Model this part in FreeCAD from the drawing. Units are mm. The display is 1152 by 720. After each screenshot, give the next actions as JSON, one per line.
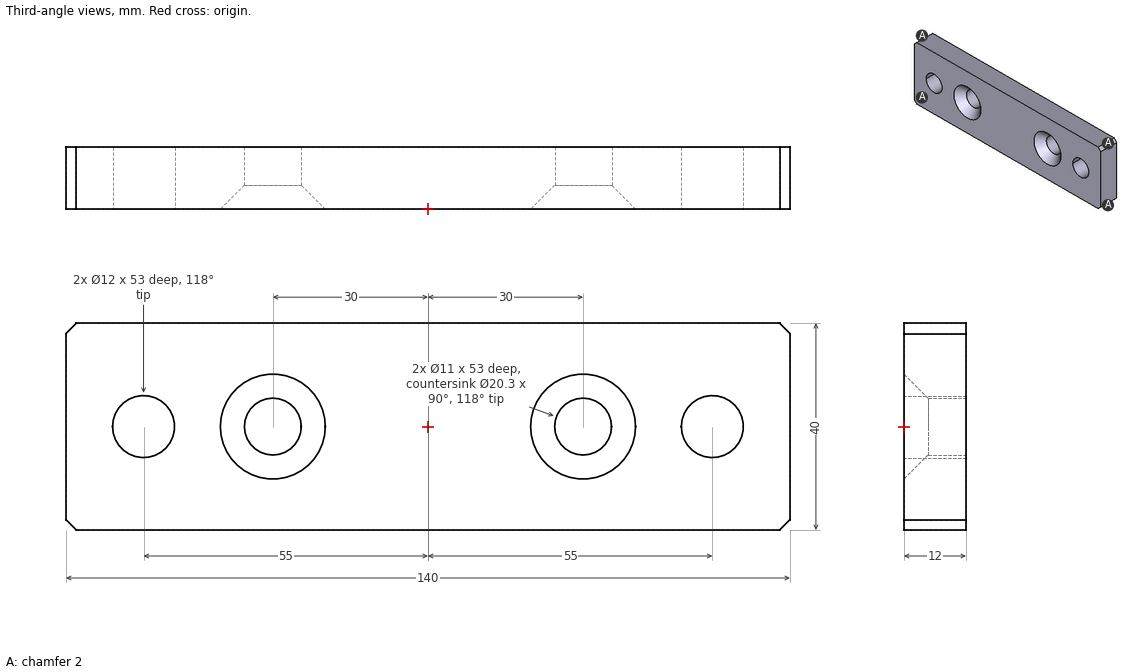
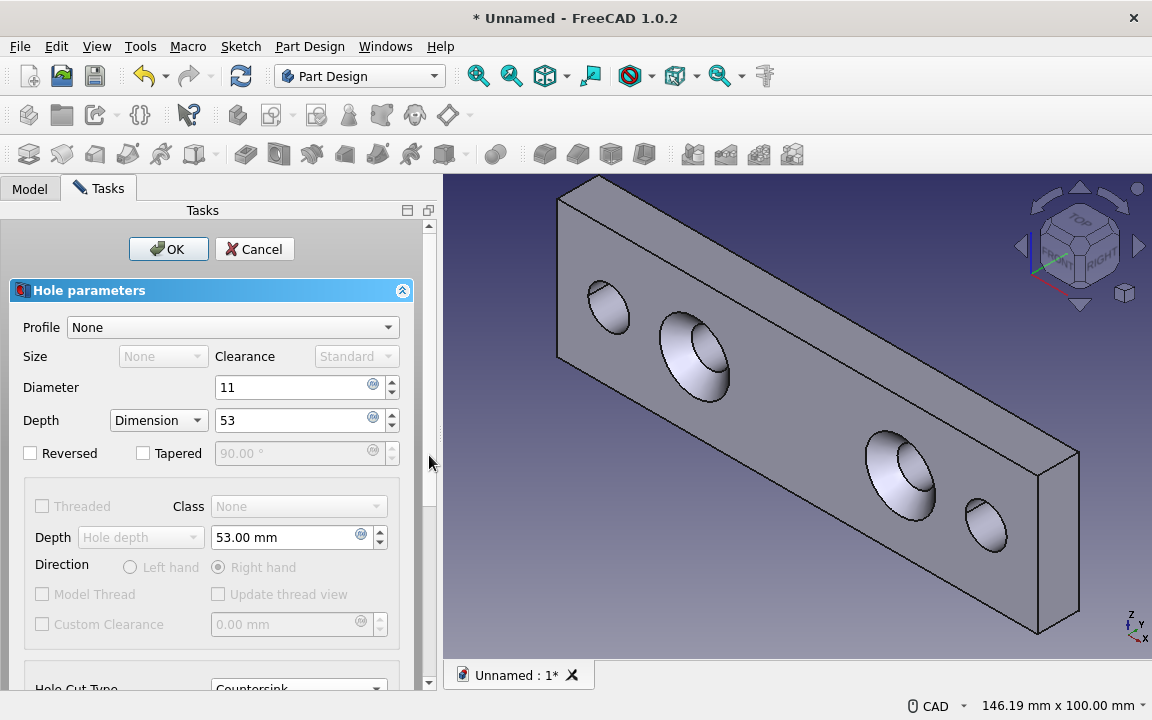
{"action": "left_click", "coordinate": [169, 249]}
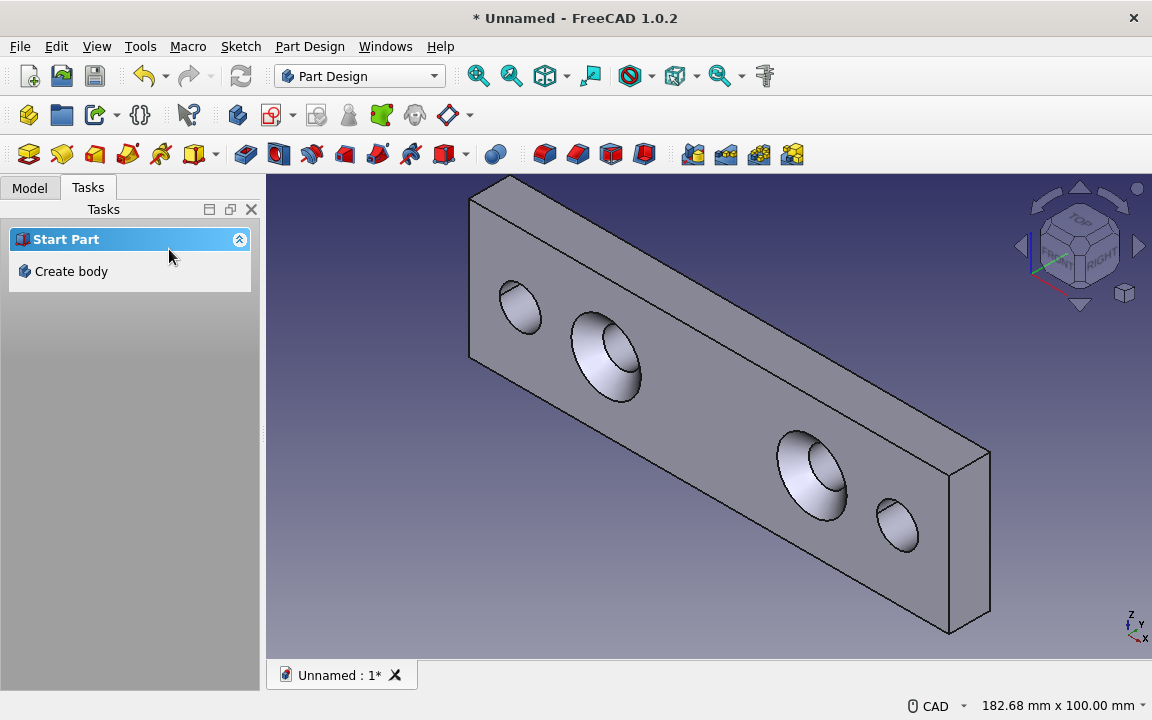
{"action": "left_click", "coordinate": [970, 463]}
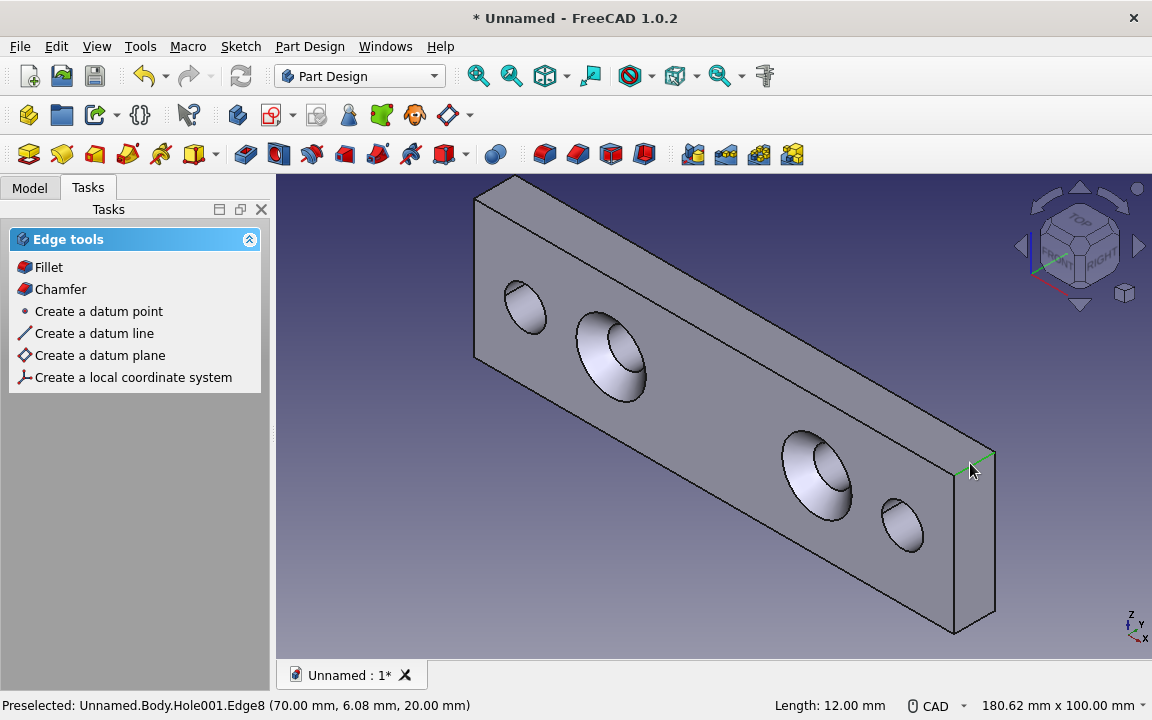
{"action": "key", "text": "2"}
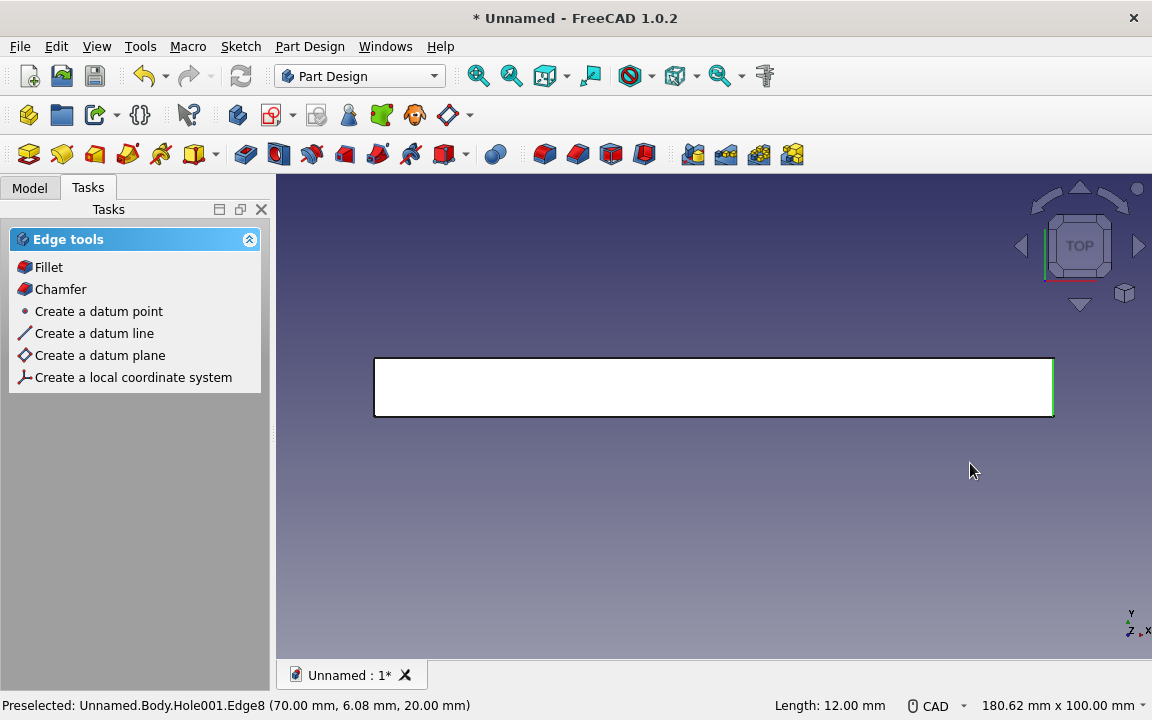
{"action": "left_click", "coordinate": [374, 386], "text": "ctrl"}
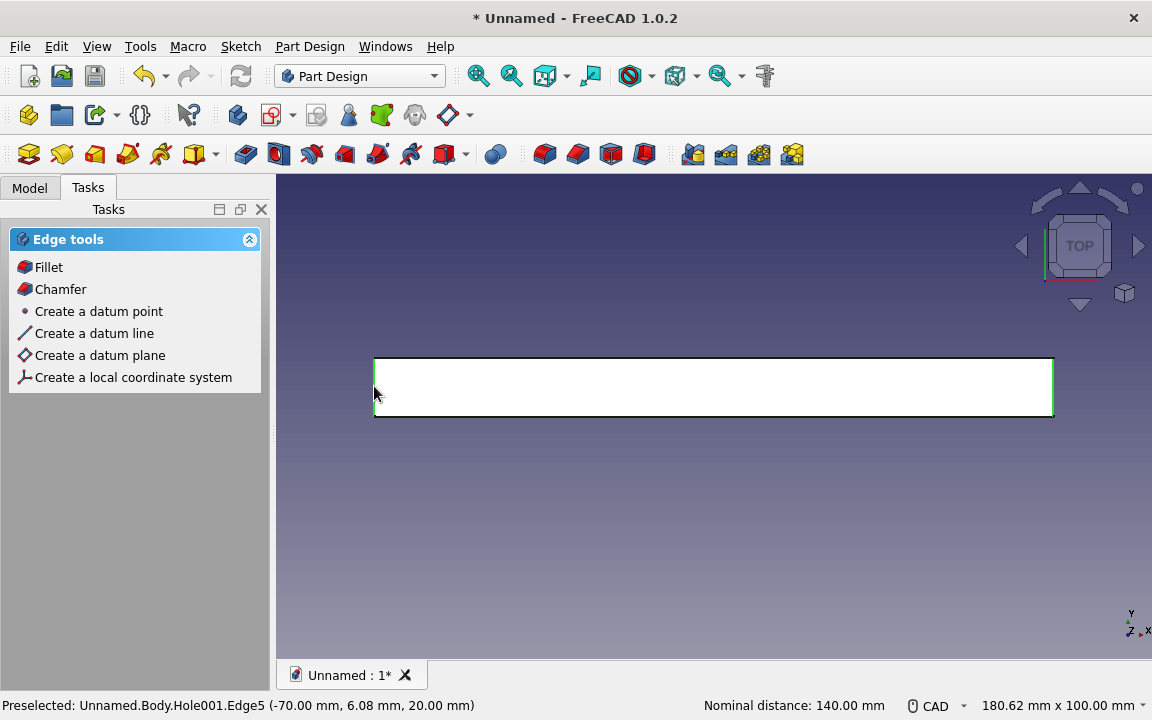
{"action": "key", "text": "0"}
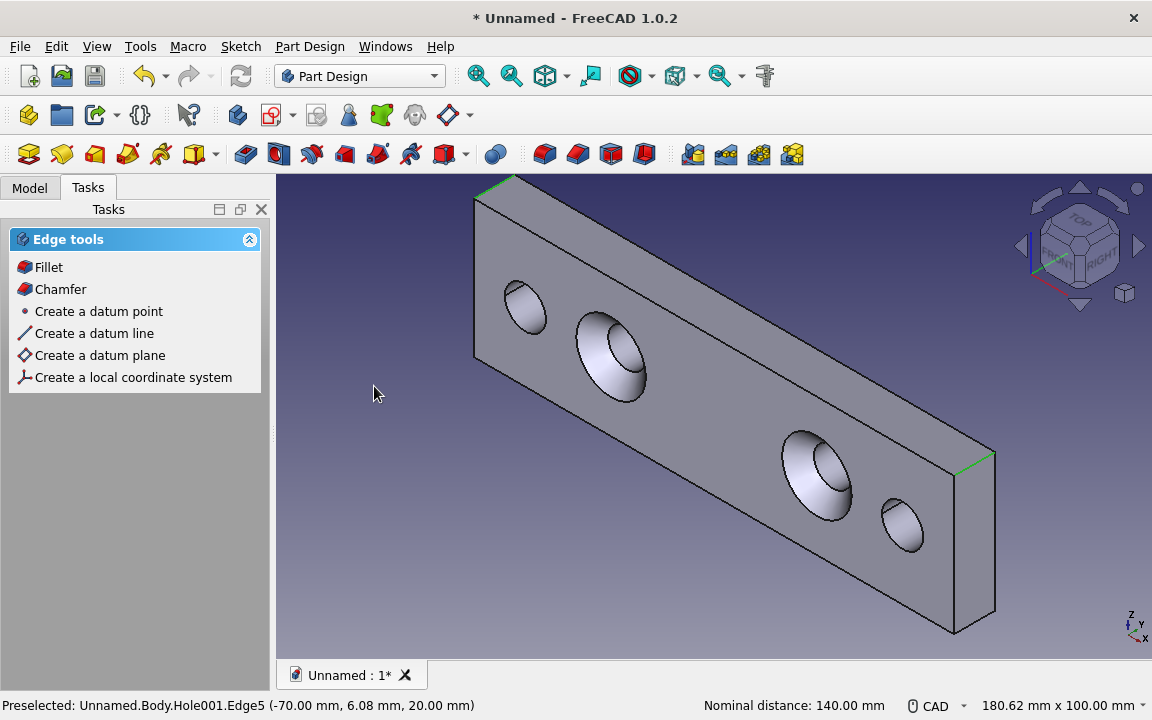
{"action": "key", "text": "1"}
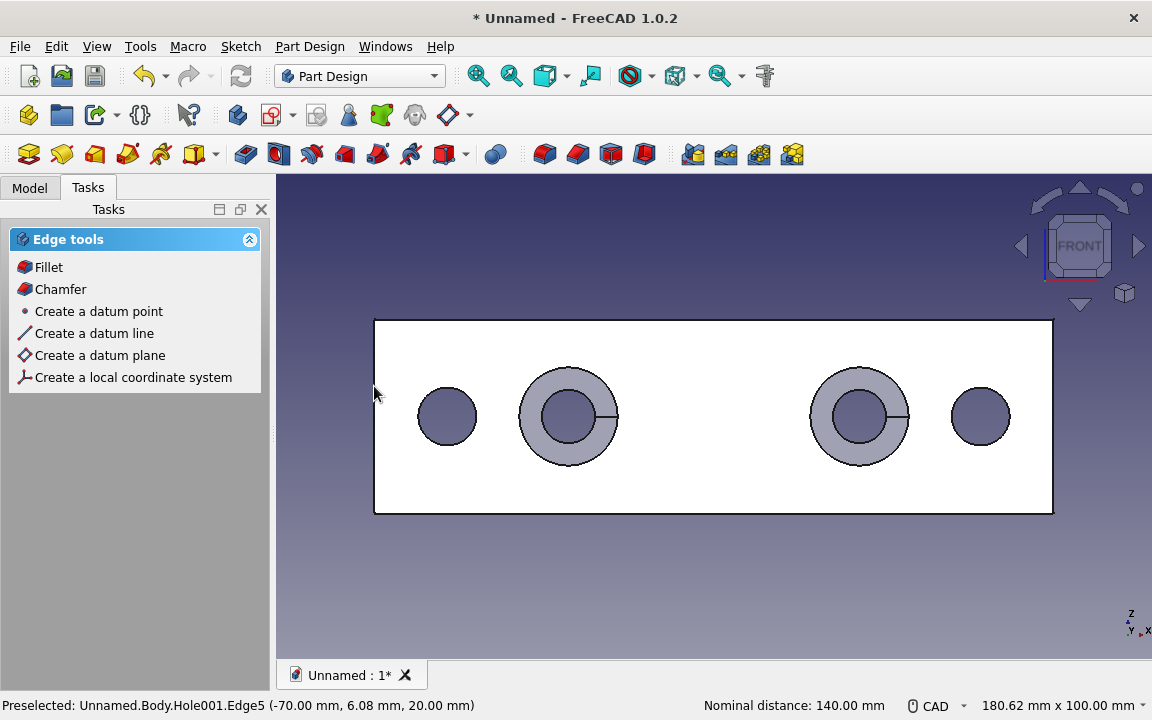
{"action": "key", "text": "3"}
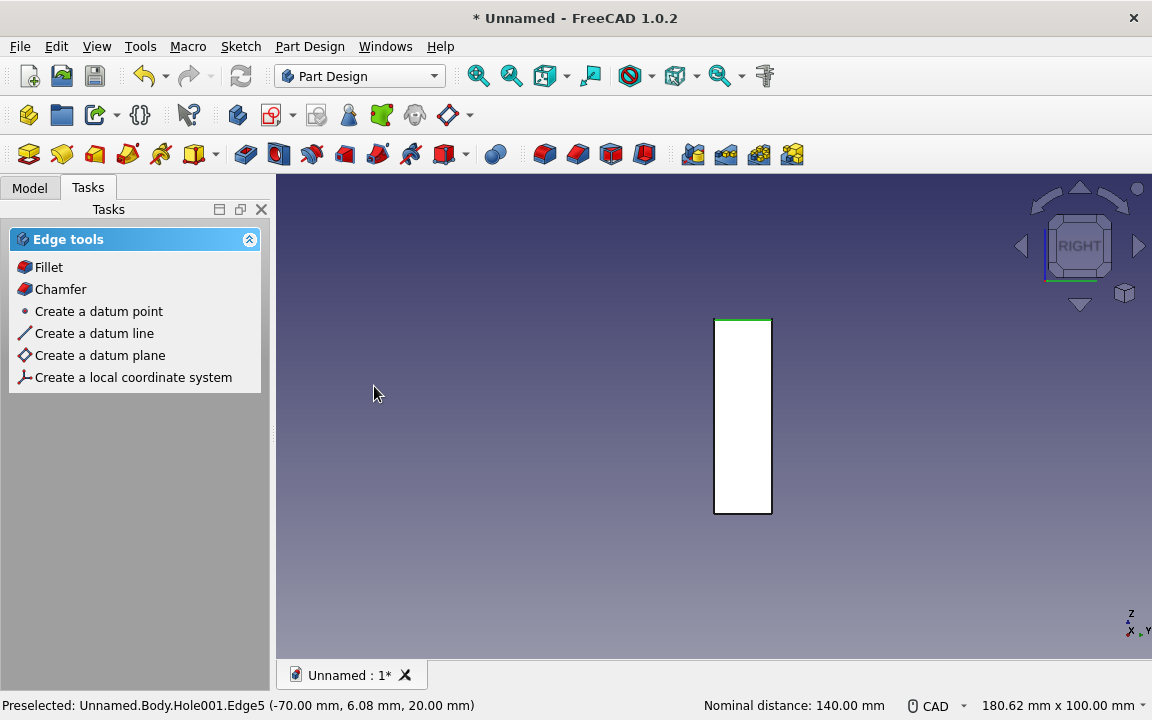
{"action": "key", "text": "v f"}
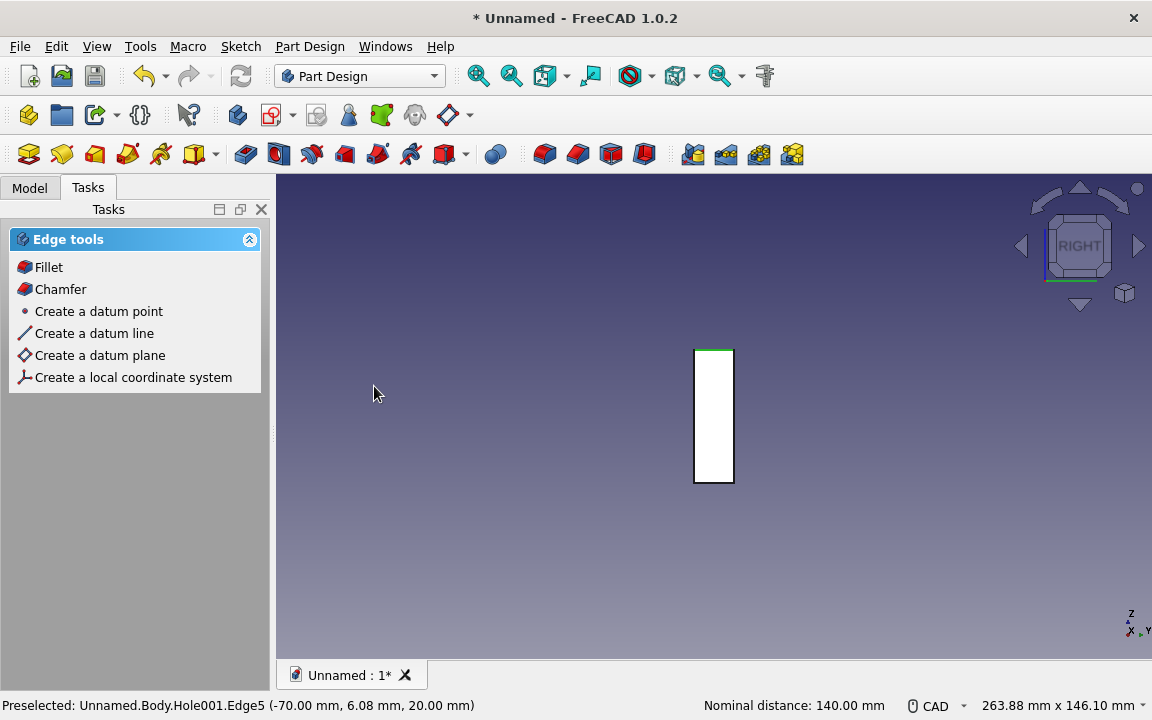
{"action": "left_click", "coordinate": [714, 482], "text": "ctrl"}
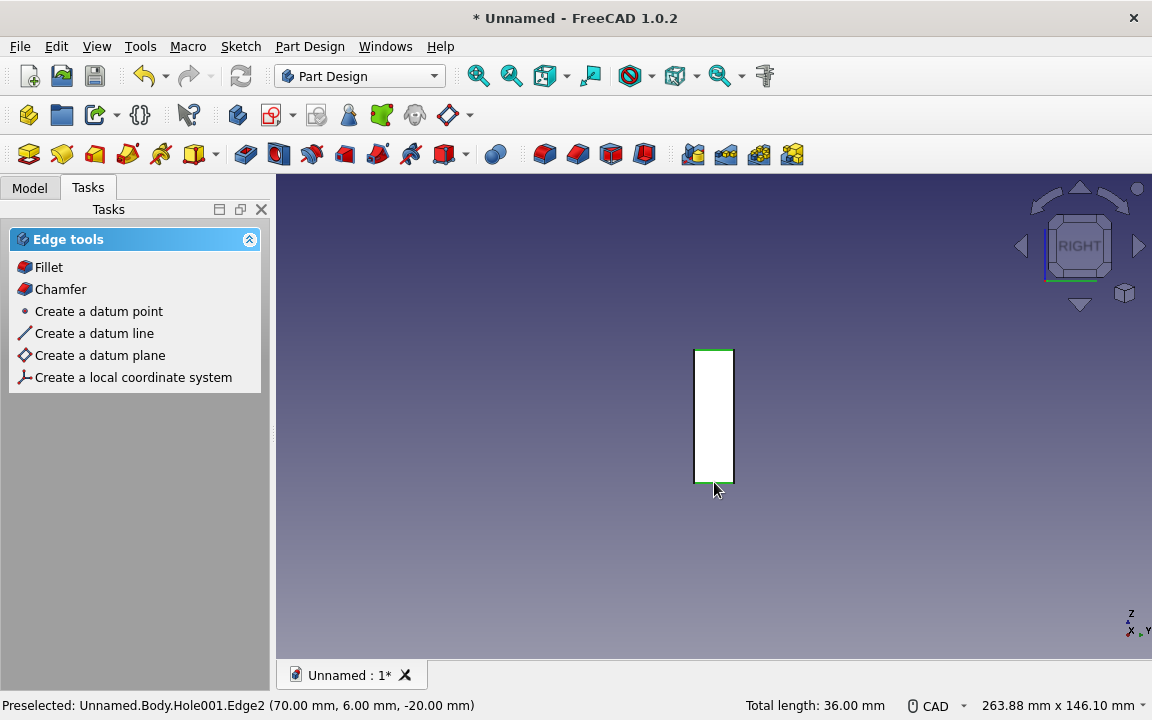
{"action": "key", "text": "5"}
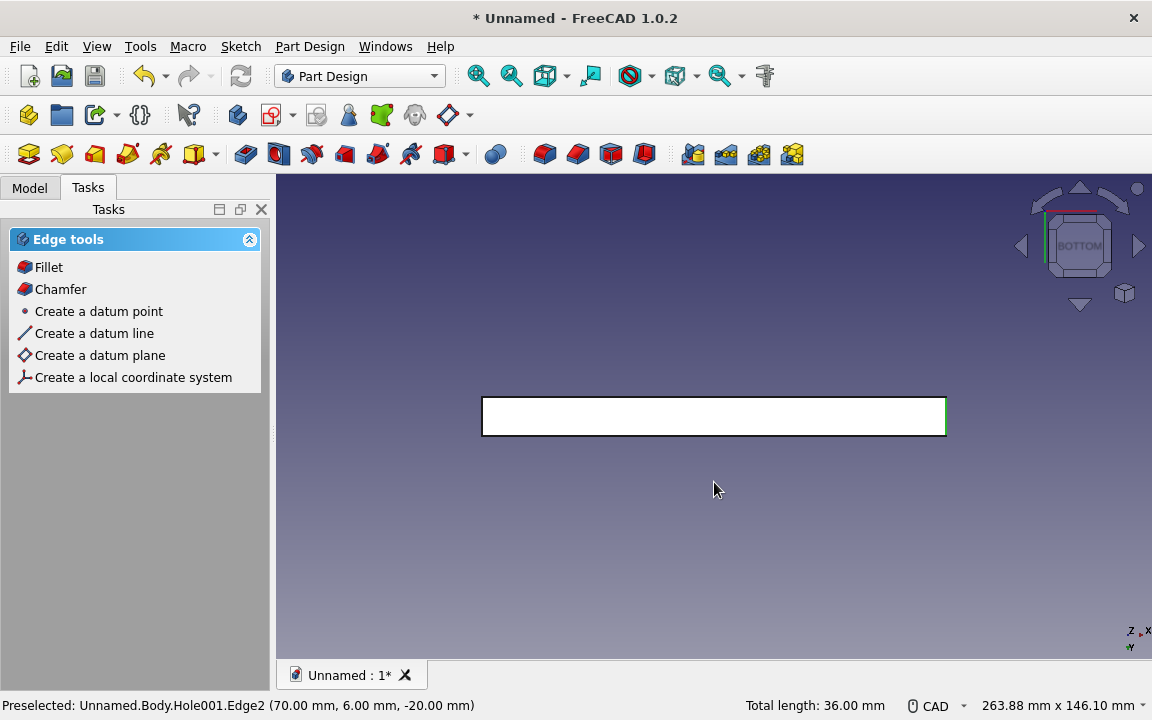
{"action": "left_click", "coordinate": [482, 415], "text": "ctrl"}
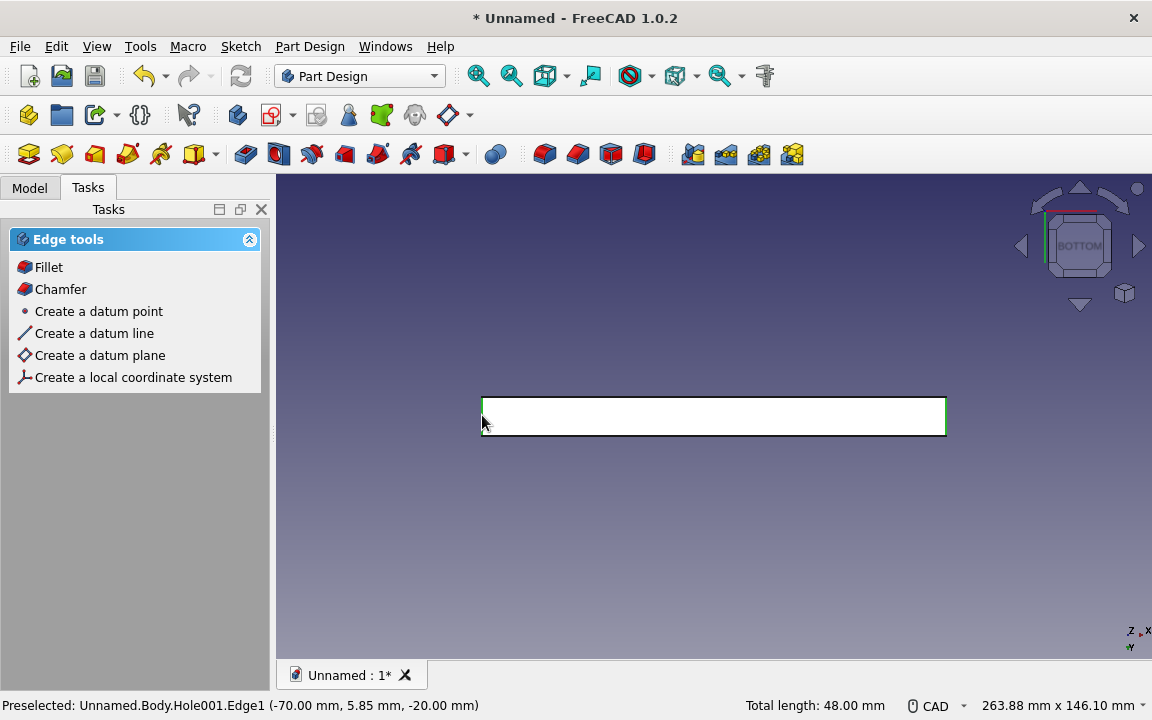
{"action": "left_click", "coordinate": [578, 154]}